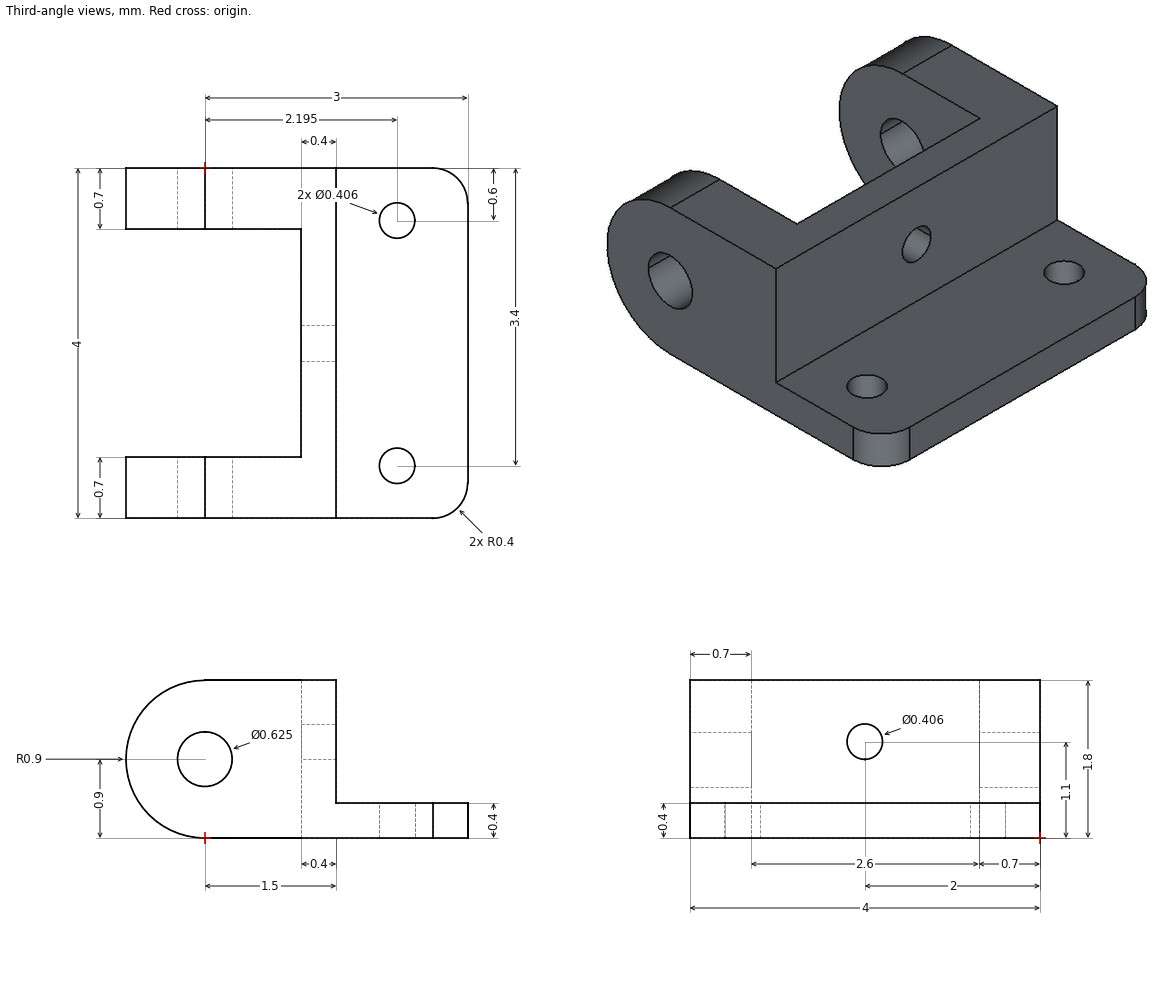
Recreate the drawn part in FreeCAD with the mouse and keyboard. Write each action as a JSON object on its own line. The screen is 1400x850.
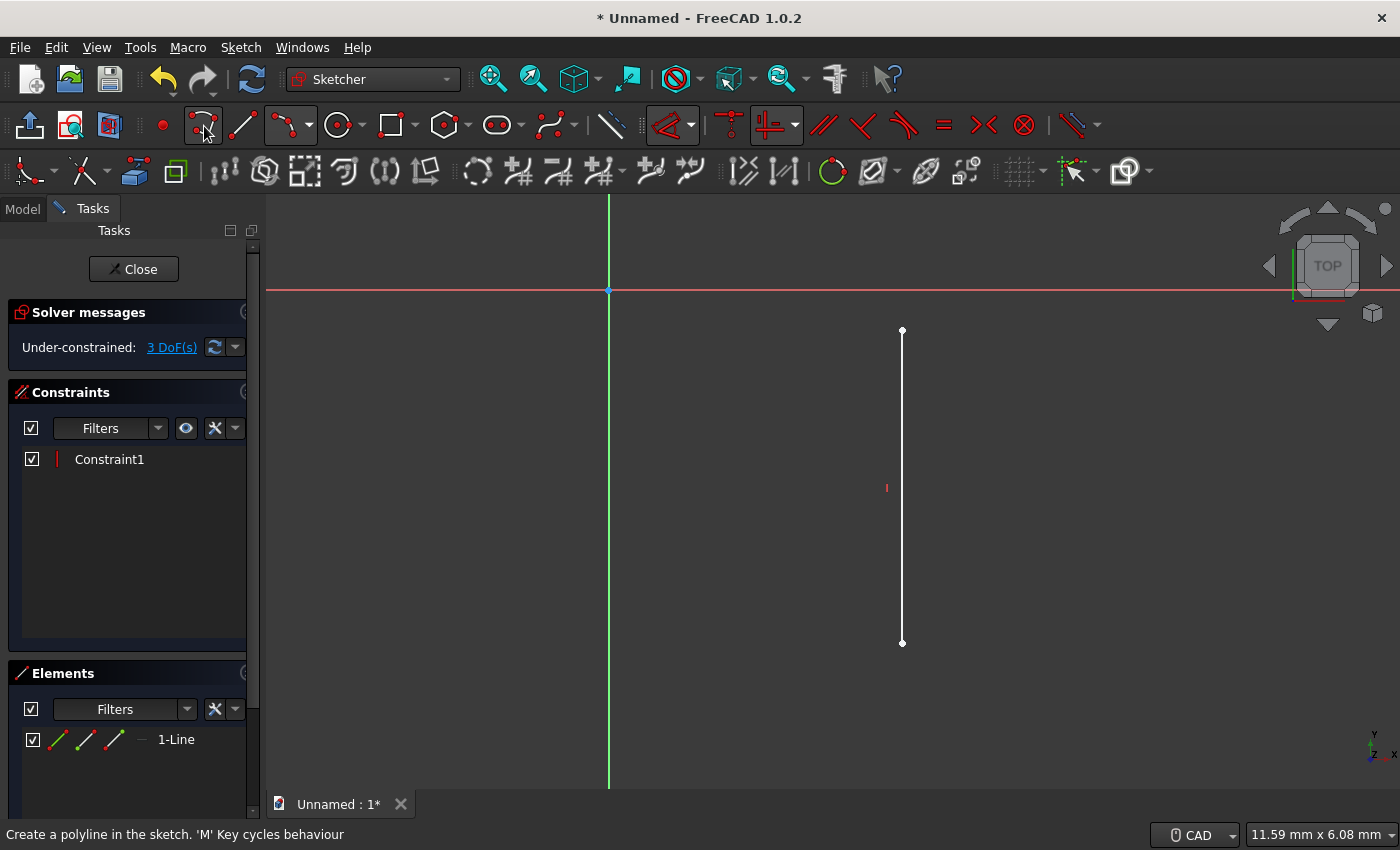
{"action": "left_click", "coordinate": [863, 290]}
{"action": "left_click", "coordinate": [609, 290]}
{"action": "left_click", "coordinate": [618, 682]}
{"action": "left_click", "coordinate": [863, 682]}
{"action": "right_click", "coordinate": [863, 682]}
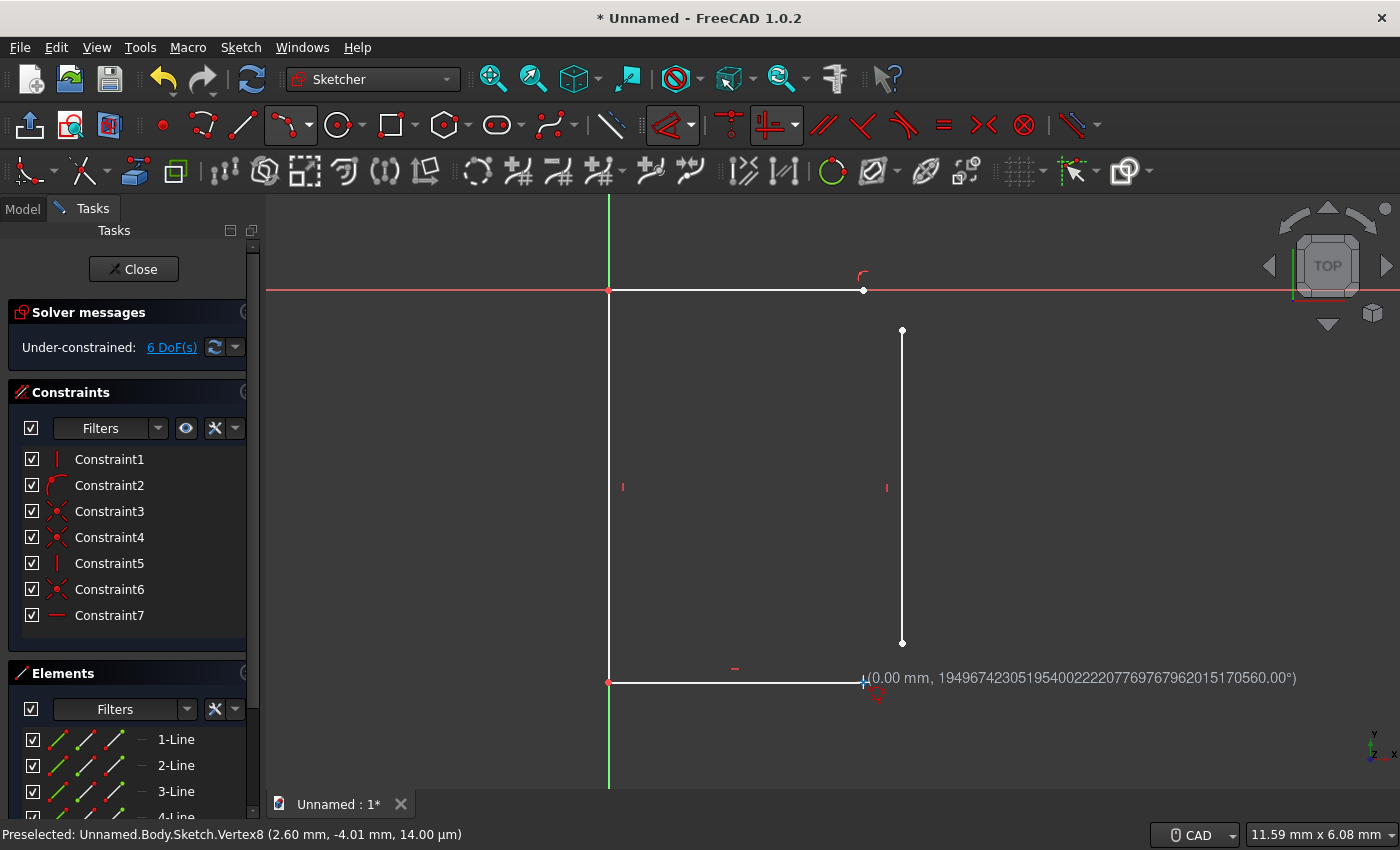
{"action": "key", "text": "g 3 a"}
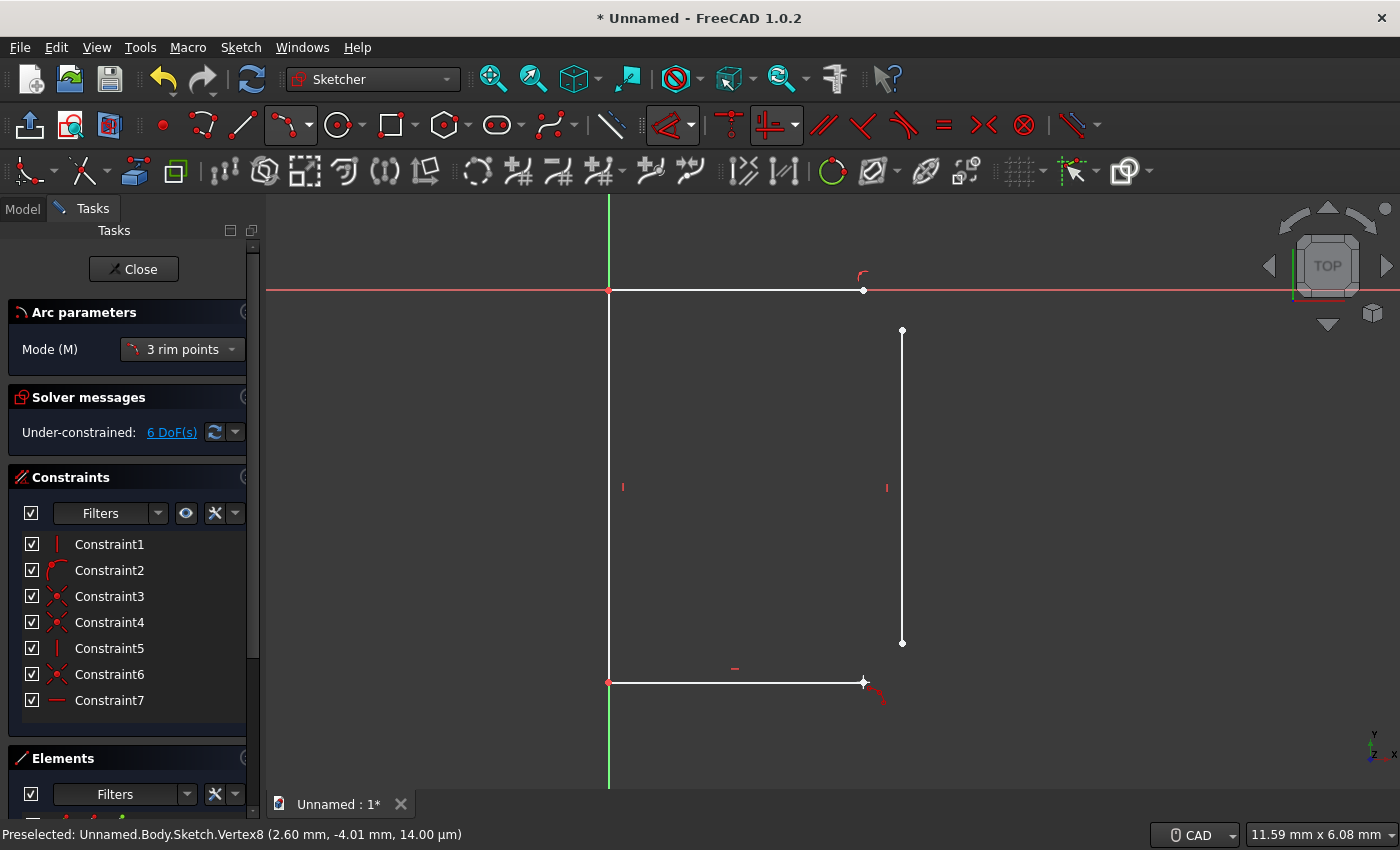
{"action": "left_click", "coordinate": [902, 331]}
{"action": "left_click", "coordinate": [863, 290]}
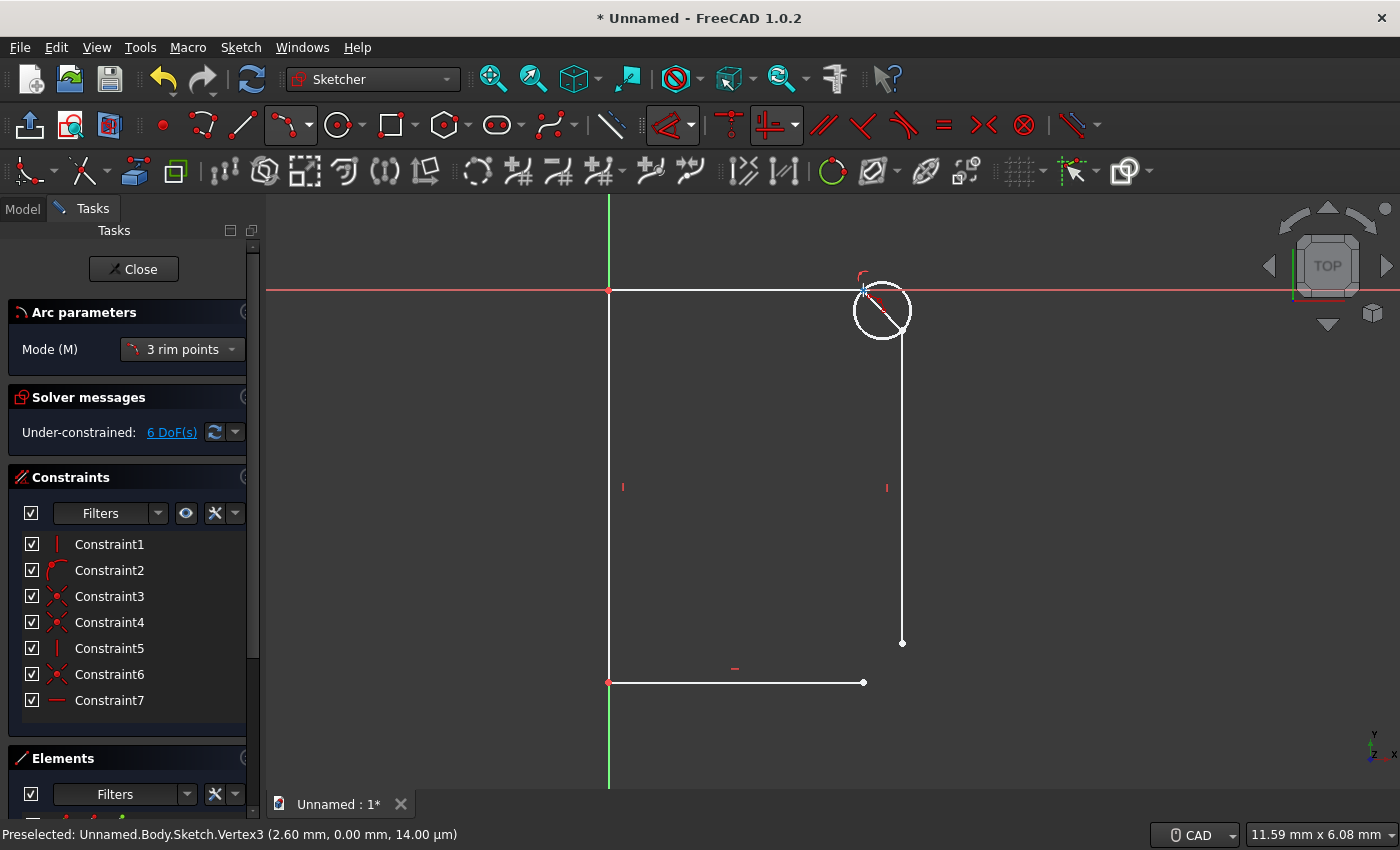
{"action": "scroll", "coordinate": [891, 302], "scroll_direction": "up", "scroll_amount": 2}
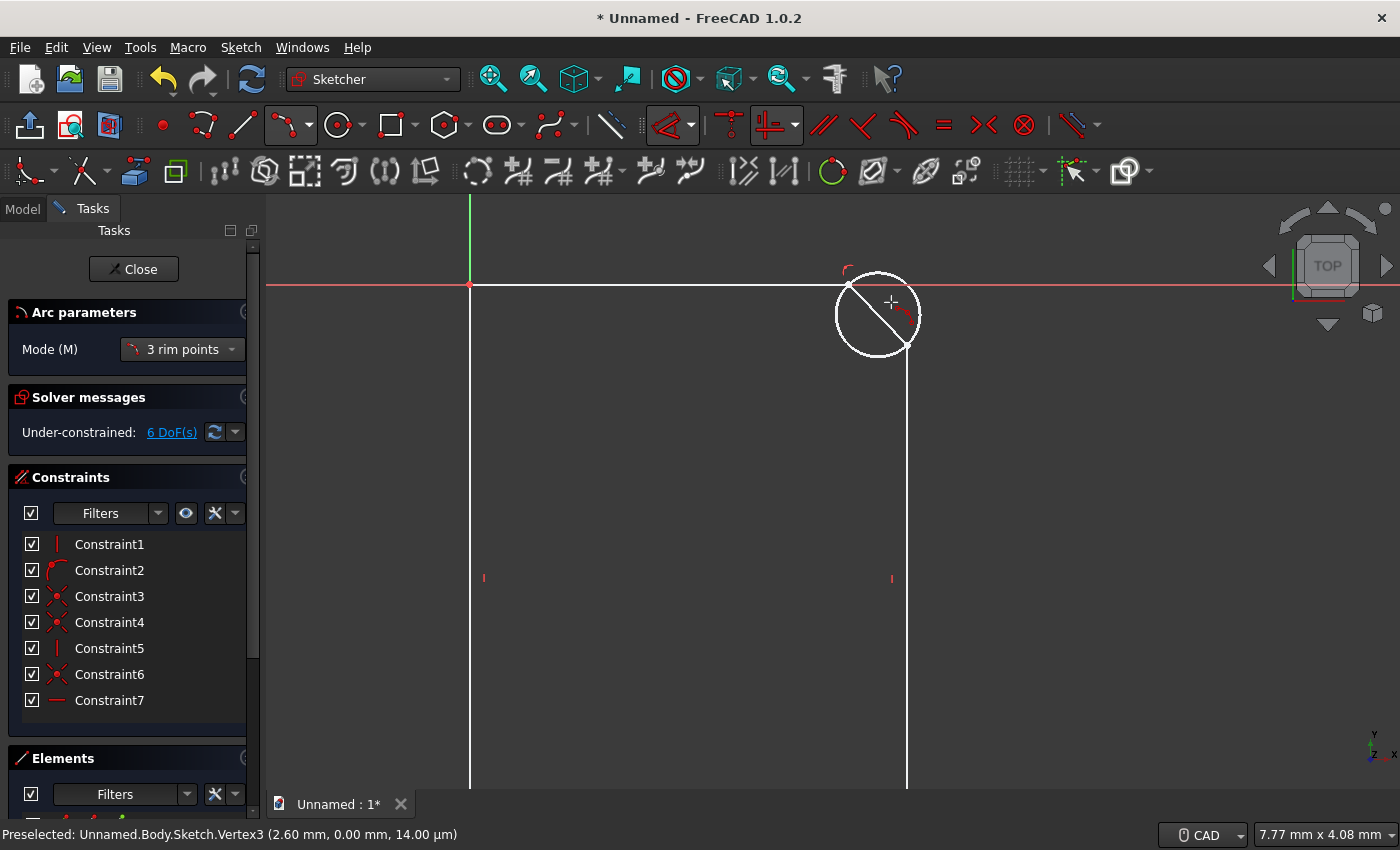
{"action": "left_click", "coordinate": [891, 302]}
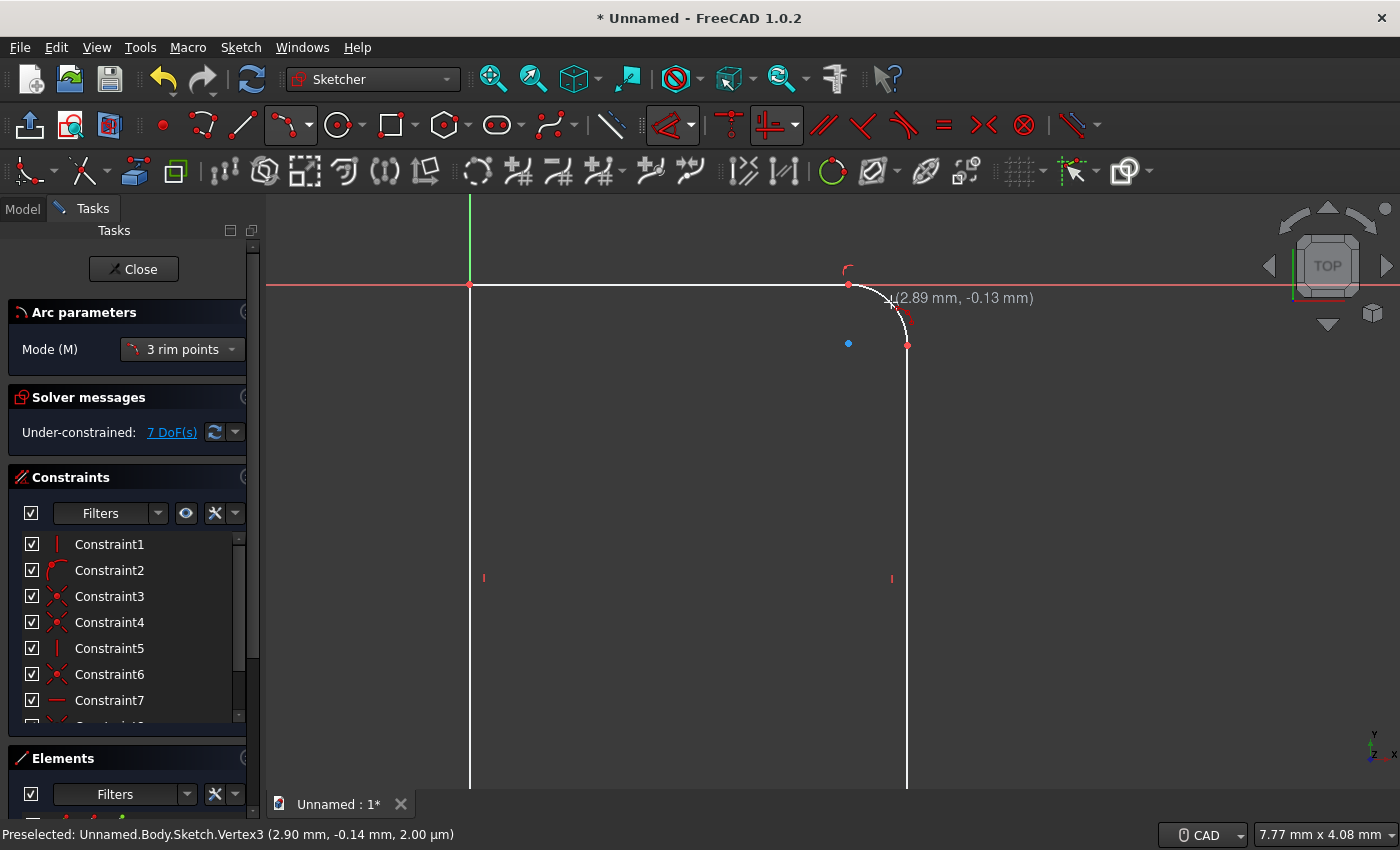
{"action": "scroll", "coordinate": [918, 319], "scroll_direction": "down", "scroll_amount": 2}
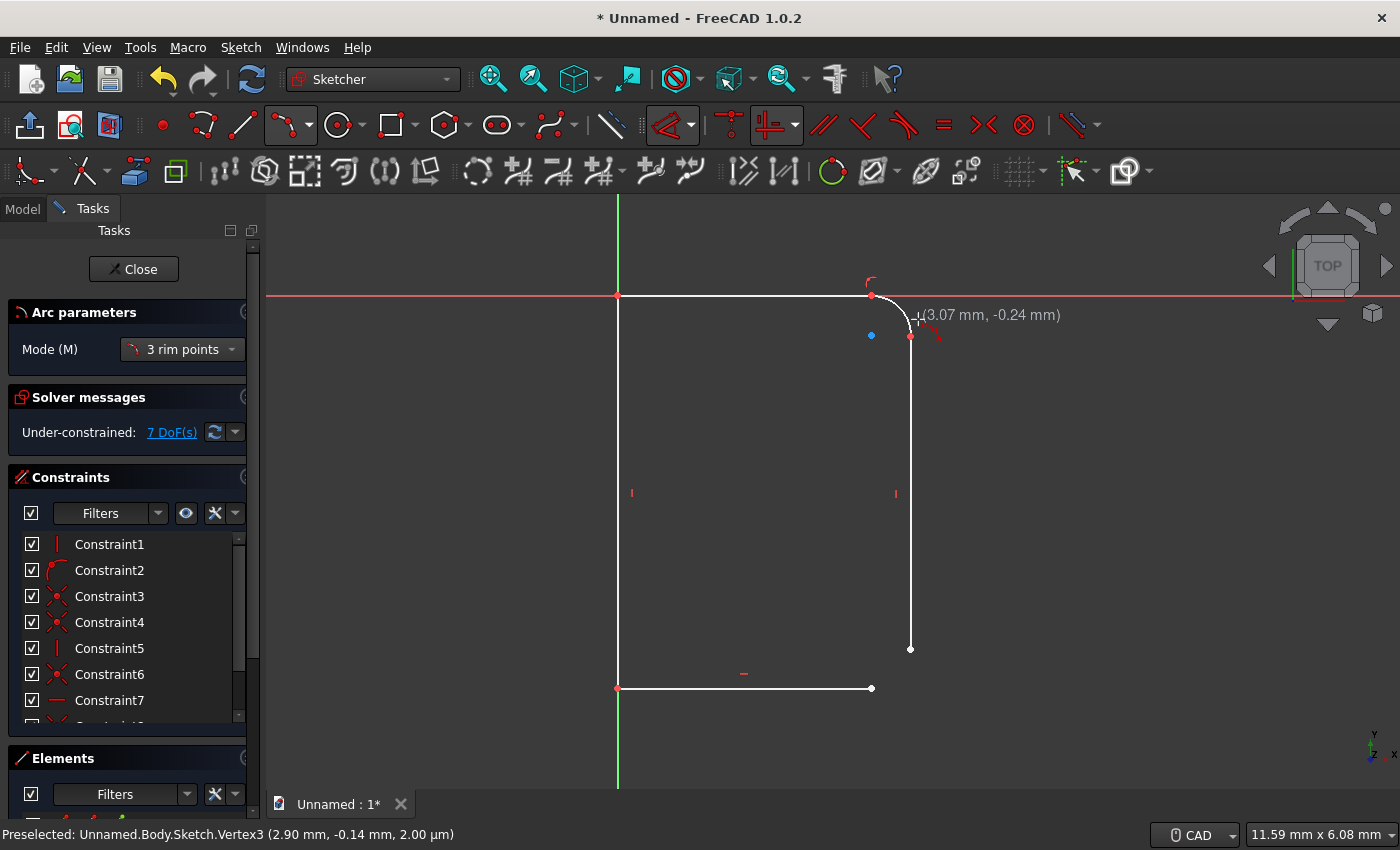
{"action": "left_click", "coordinate": [872, 689]}
{"action": "left_click", "coordinate": [911, 650]}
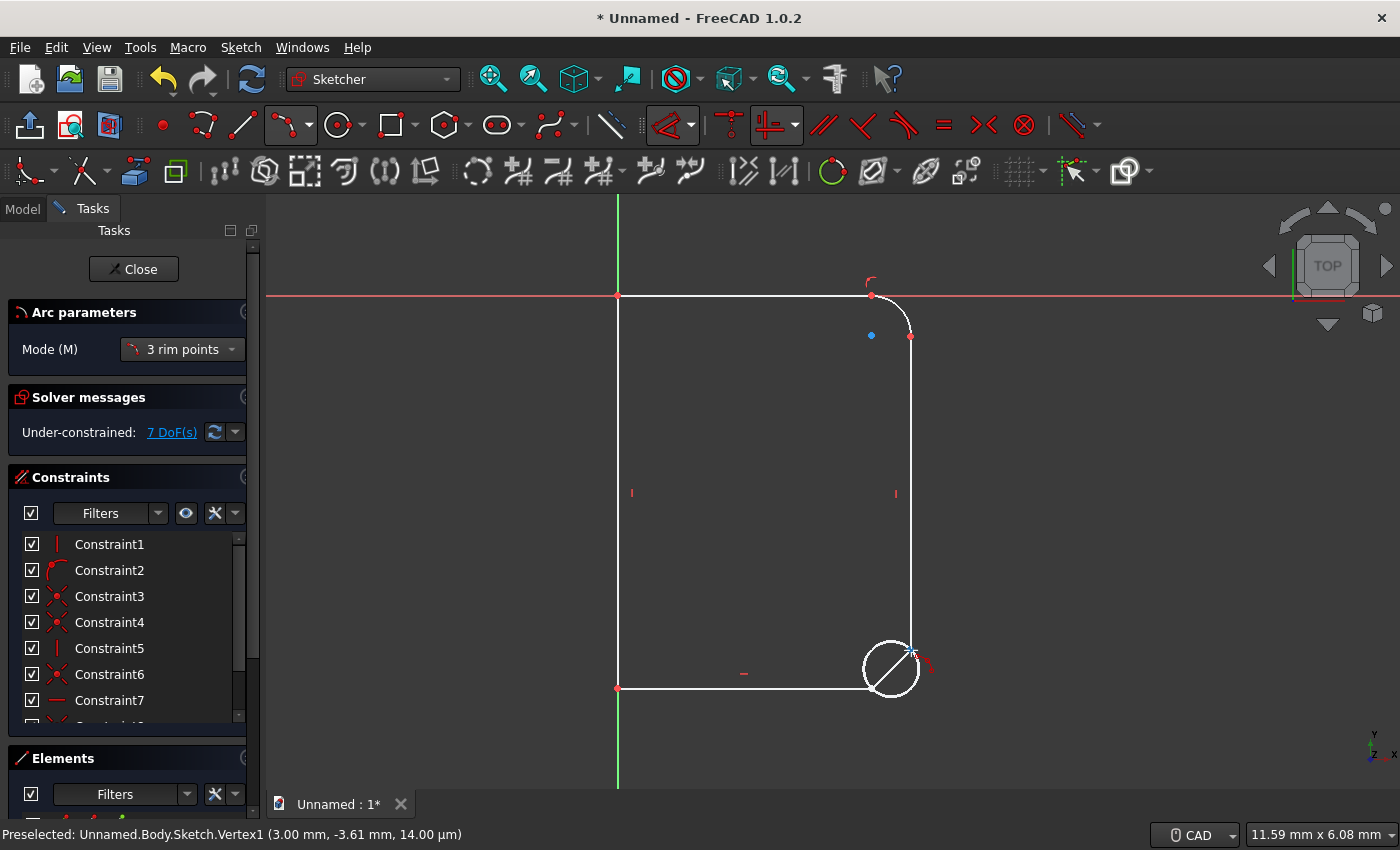
{"action": "scroll", "coordinate": [900, 676], "scroll_direction": "up", "scroll_amount": 2}